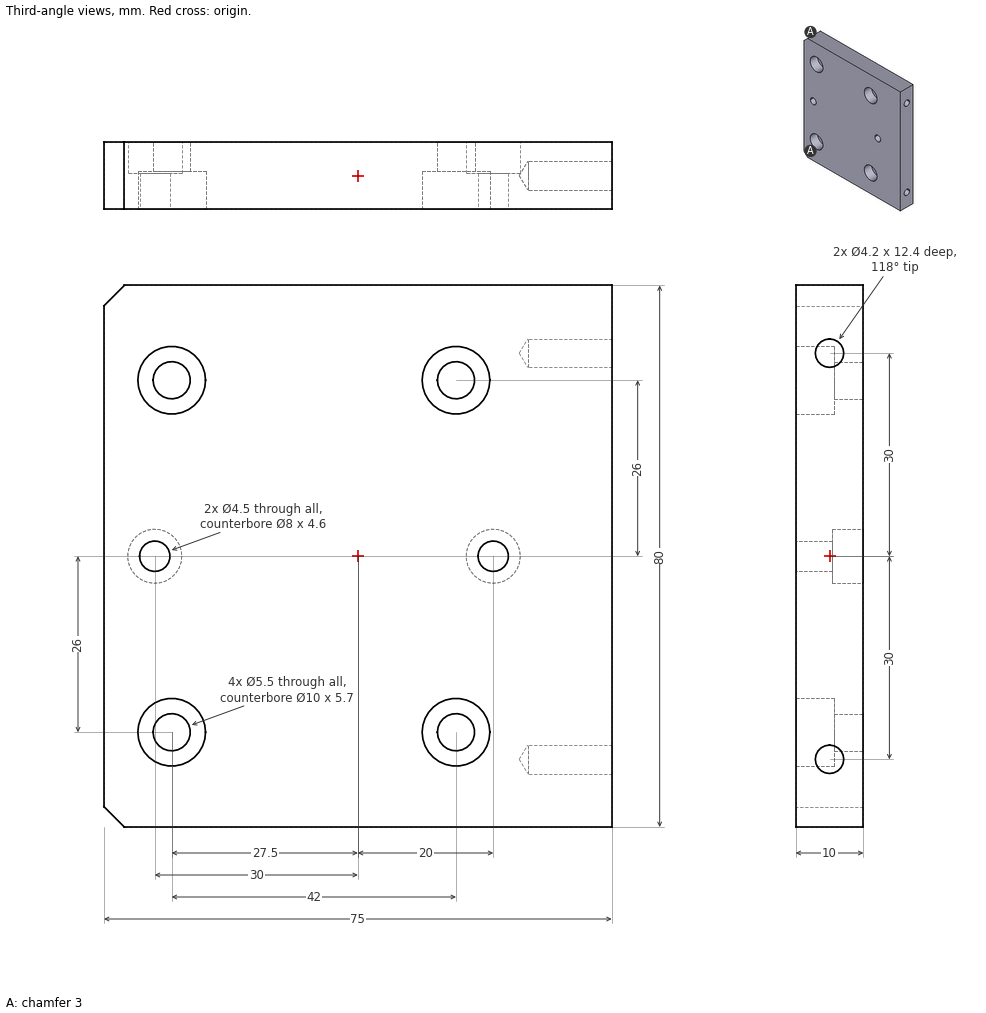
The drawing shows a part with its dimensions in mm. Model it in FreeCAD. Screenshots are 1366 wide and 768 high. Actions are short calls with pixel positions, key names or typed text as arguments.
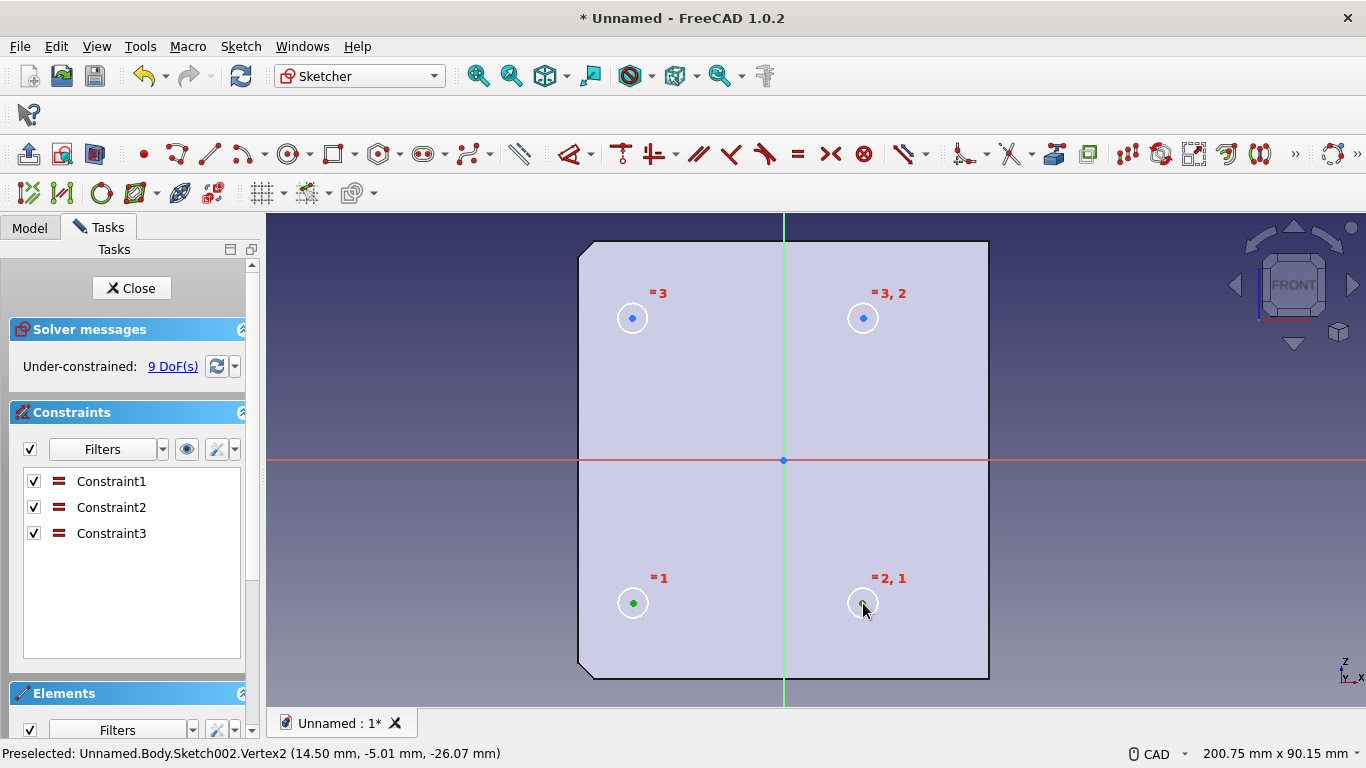
click(676, 154)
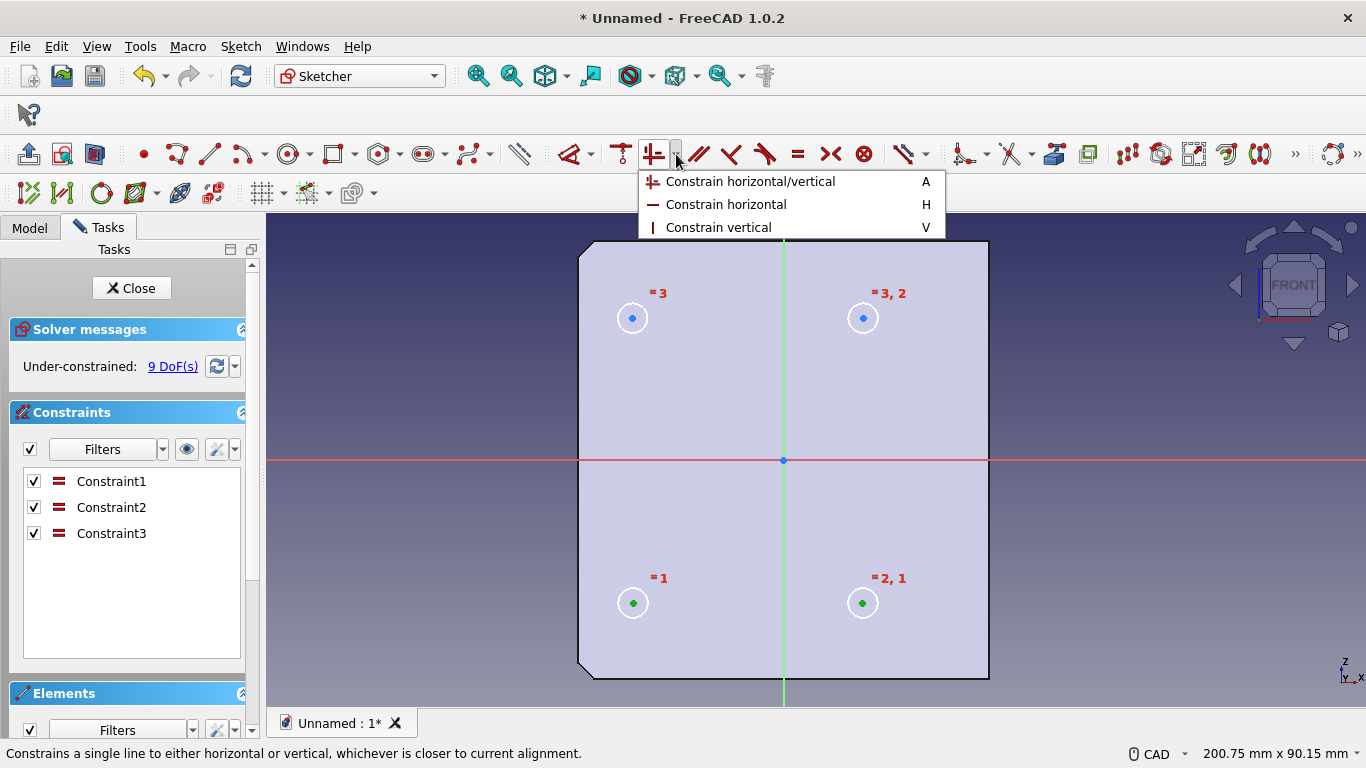
click(792, 204)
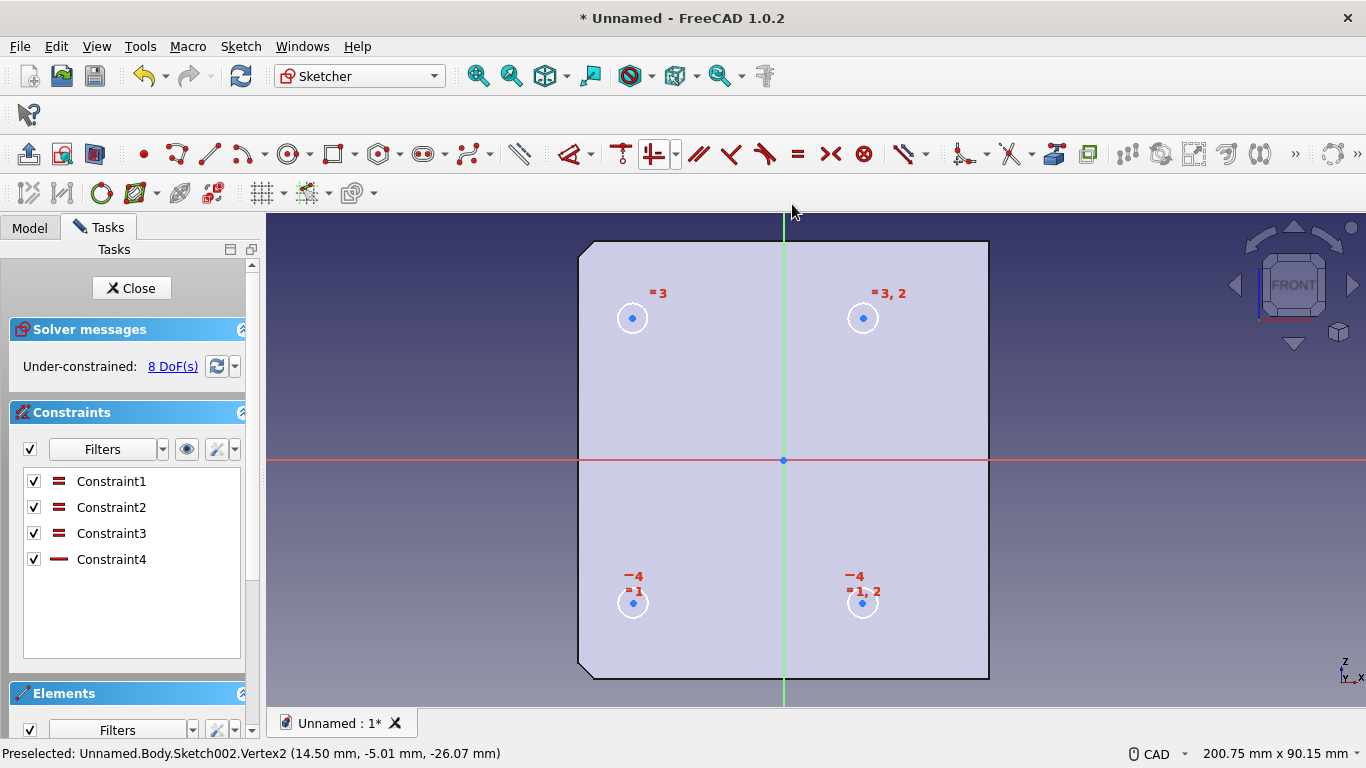
click(863, 603)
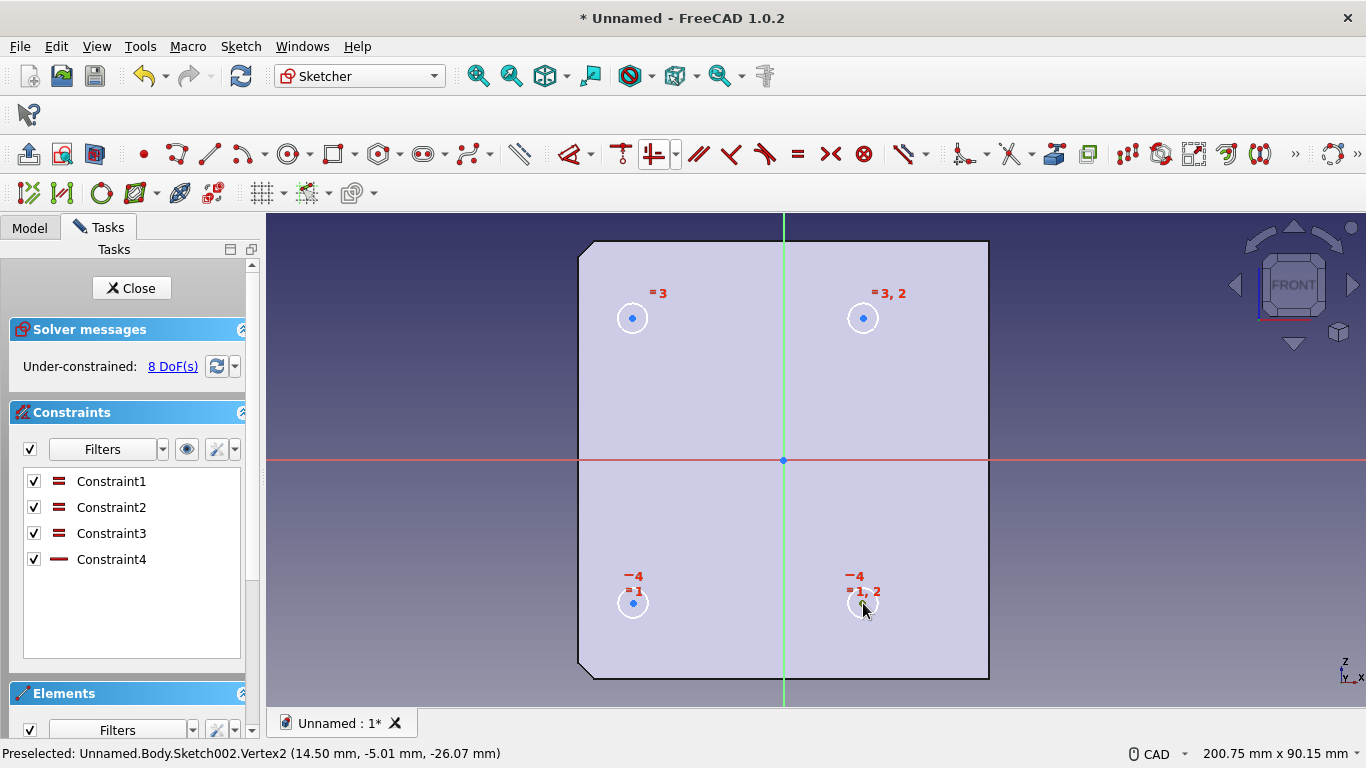
click(863, 318)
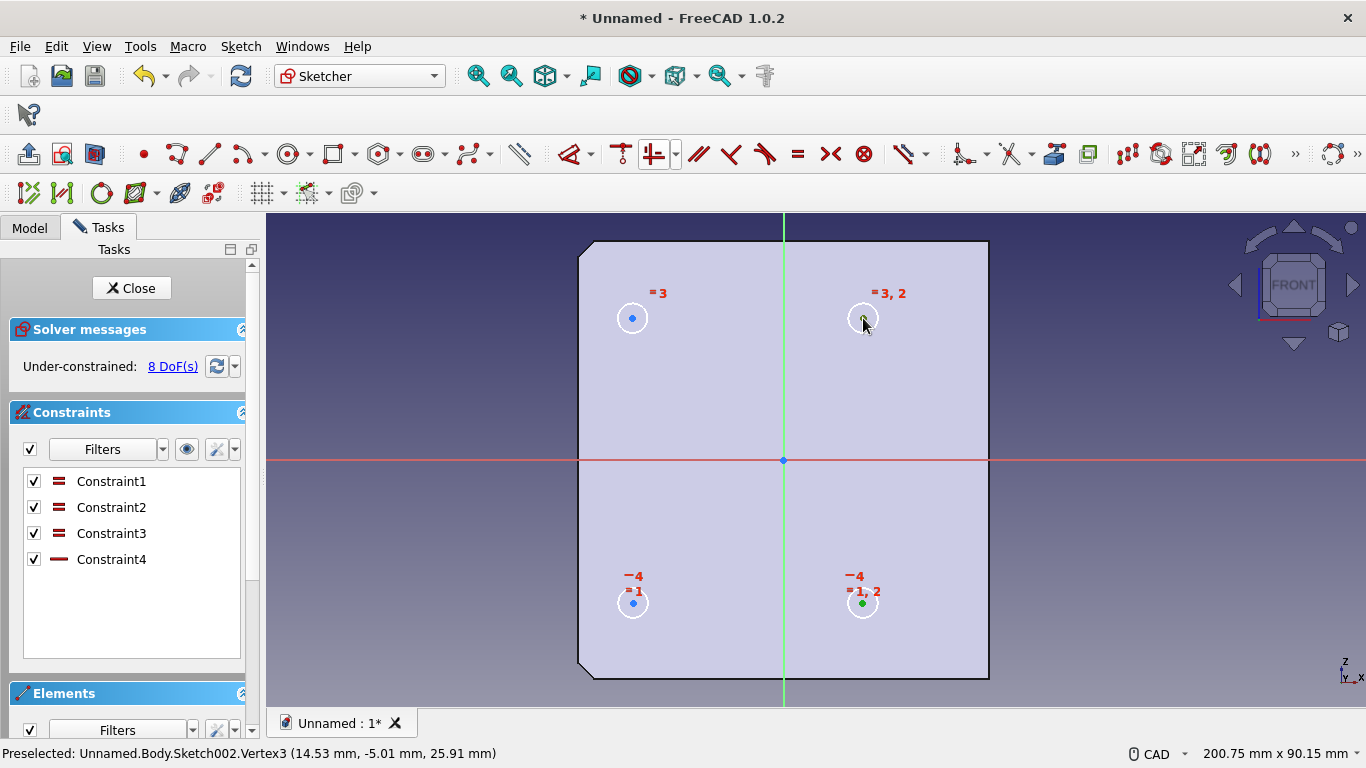
click(676, 154)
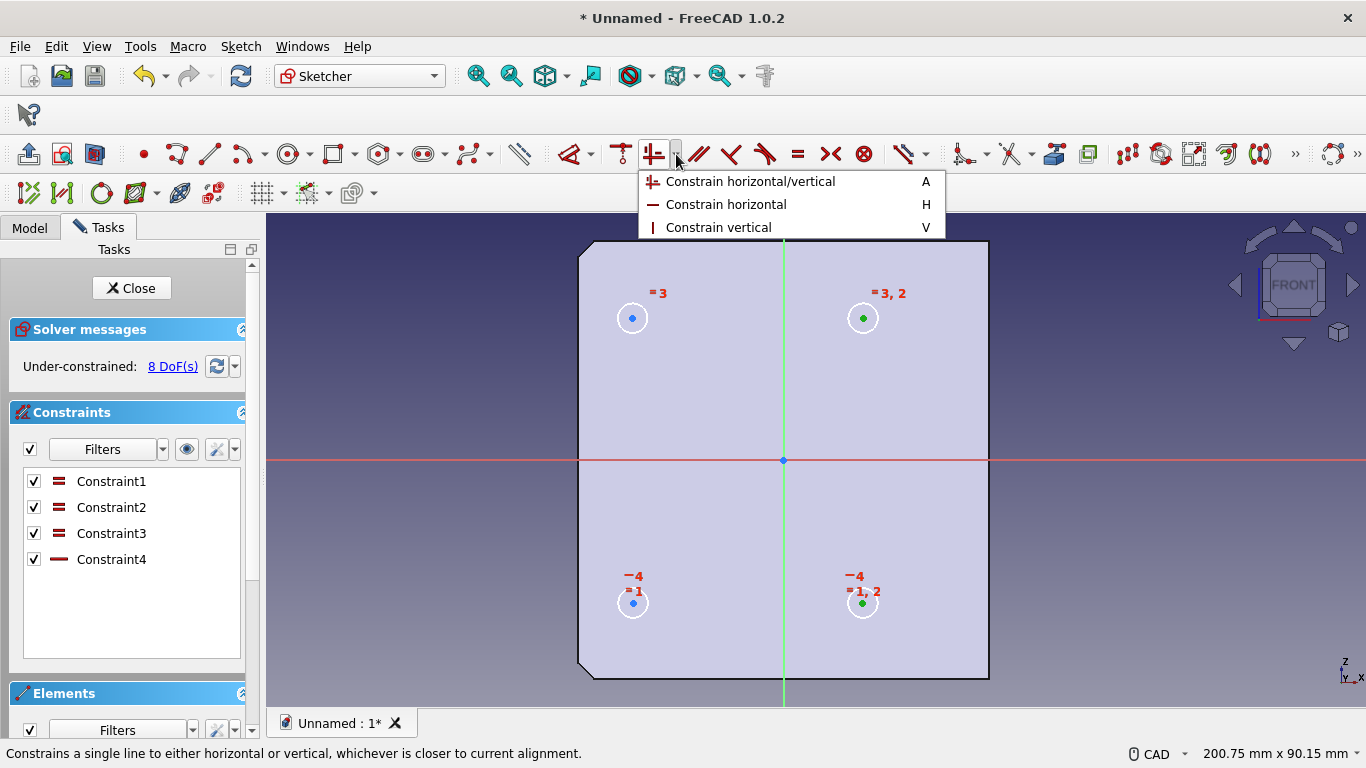
click(792, 228)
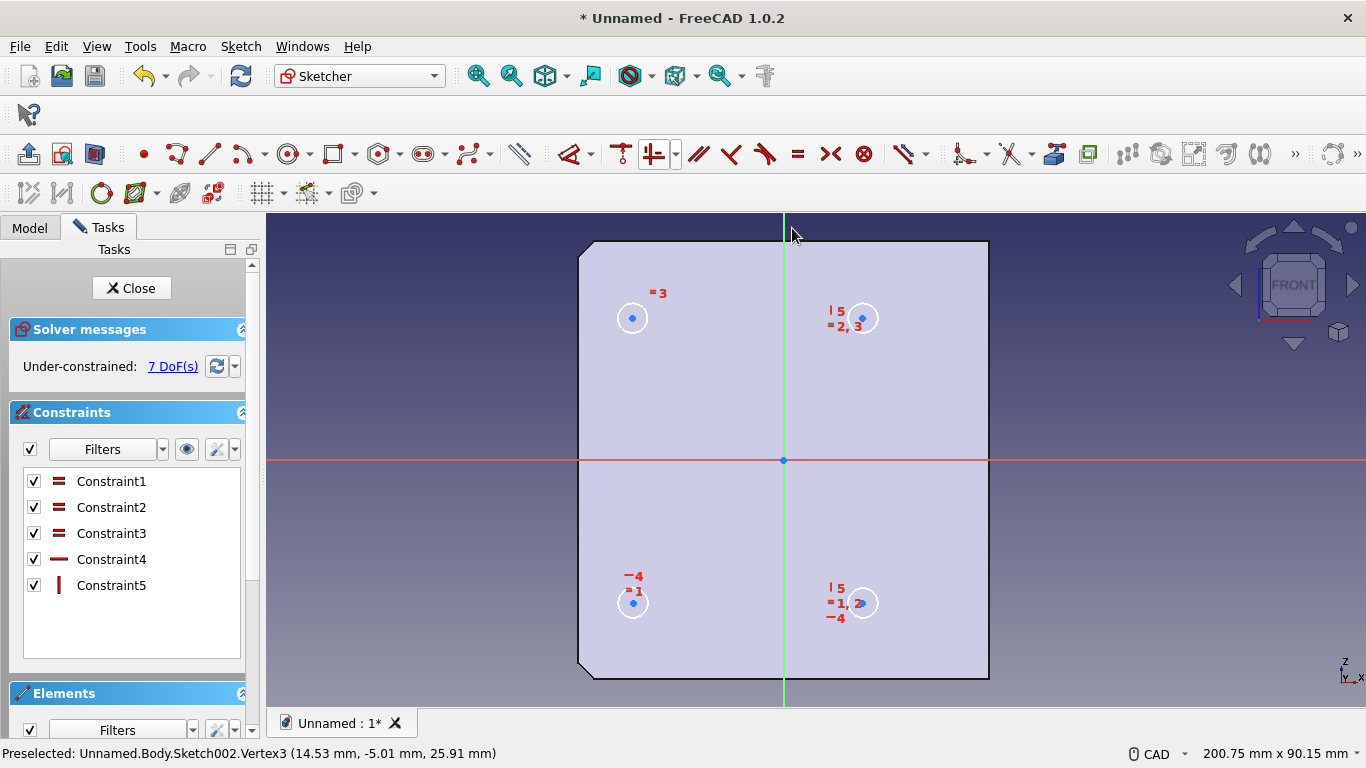
click(633, 603)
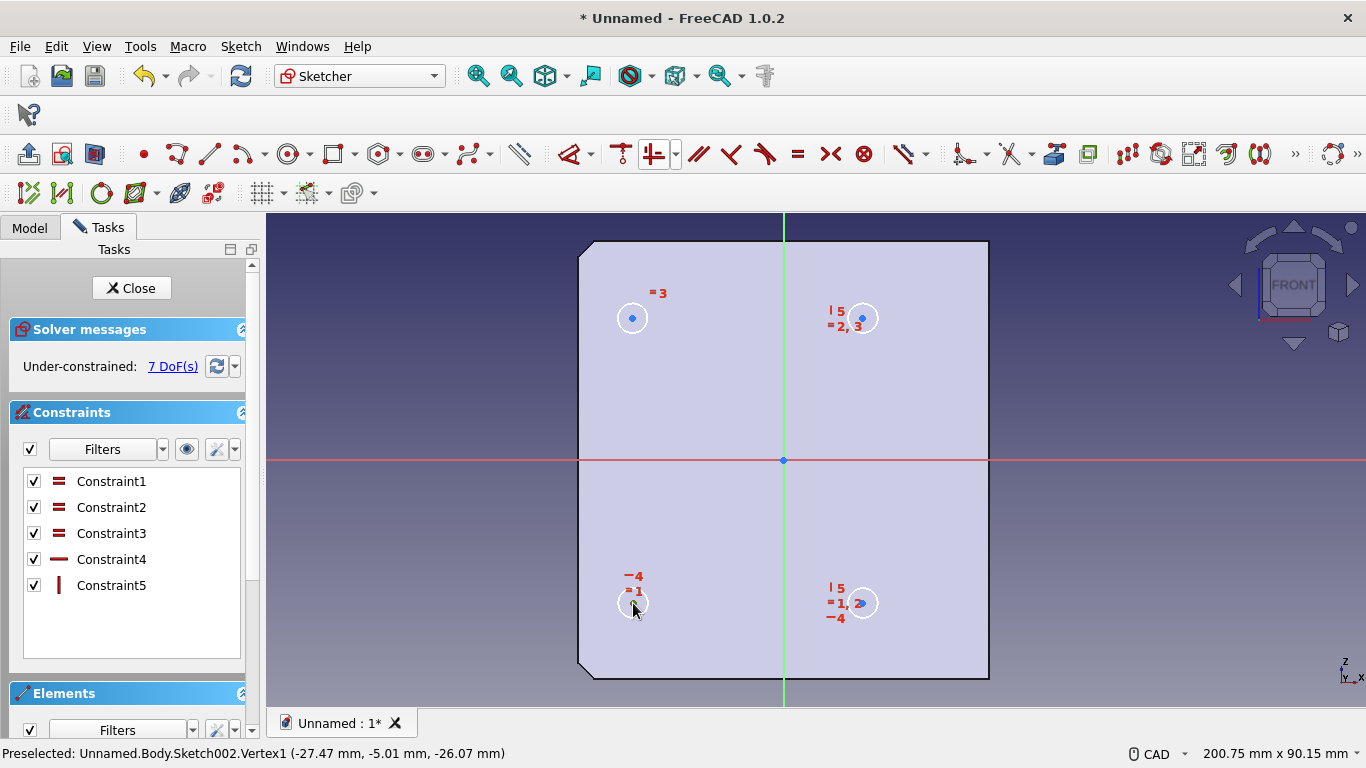
click(633, 318)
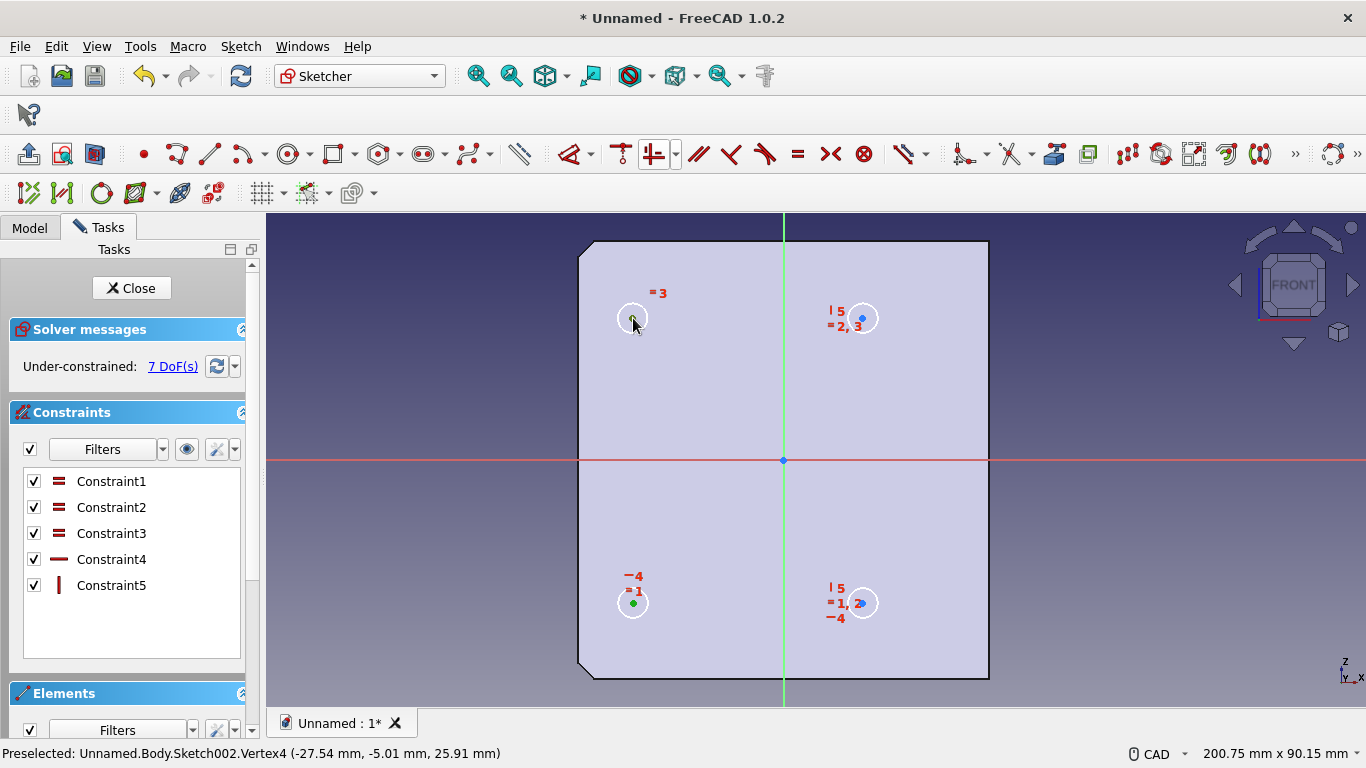
click(676, 154)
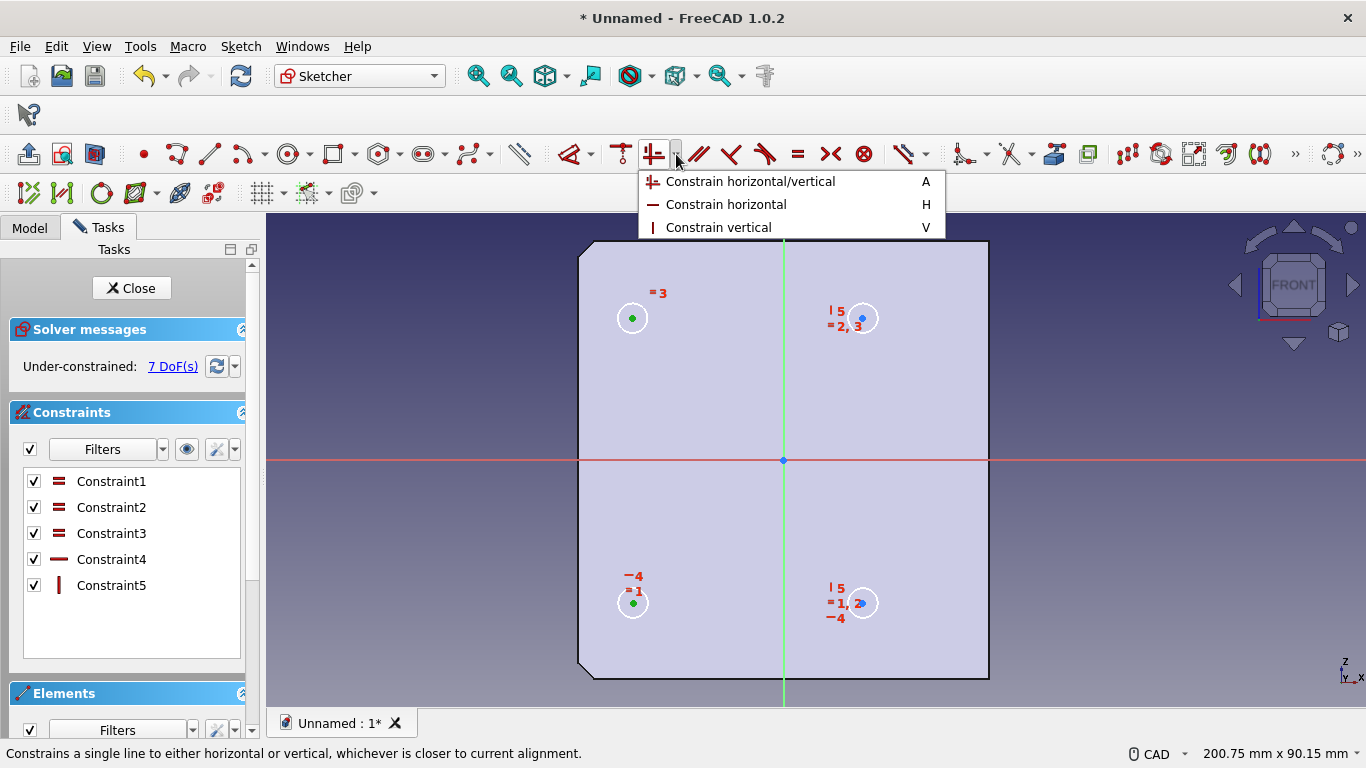
click(792, 228)